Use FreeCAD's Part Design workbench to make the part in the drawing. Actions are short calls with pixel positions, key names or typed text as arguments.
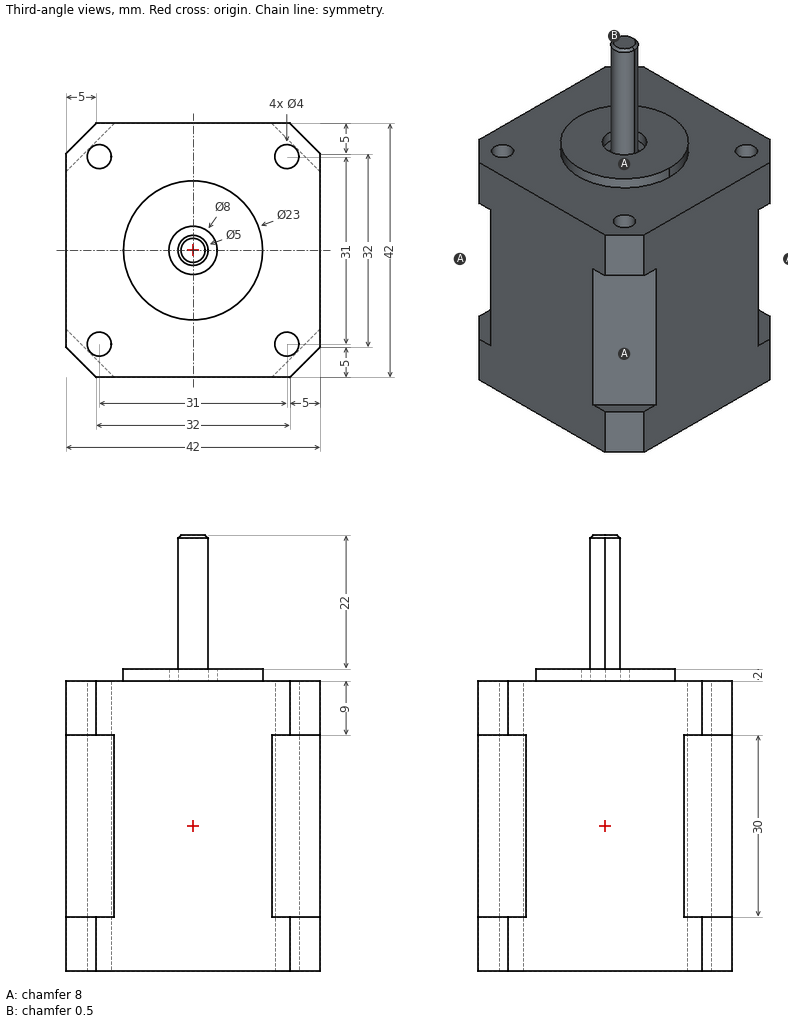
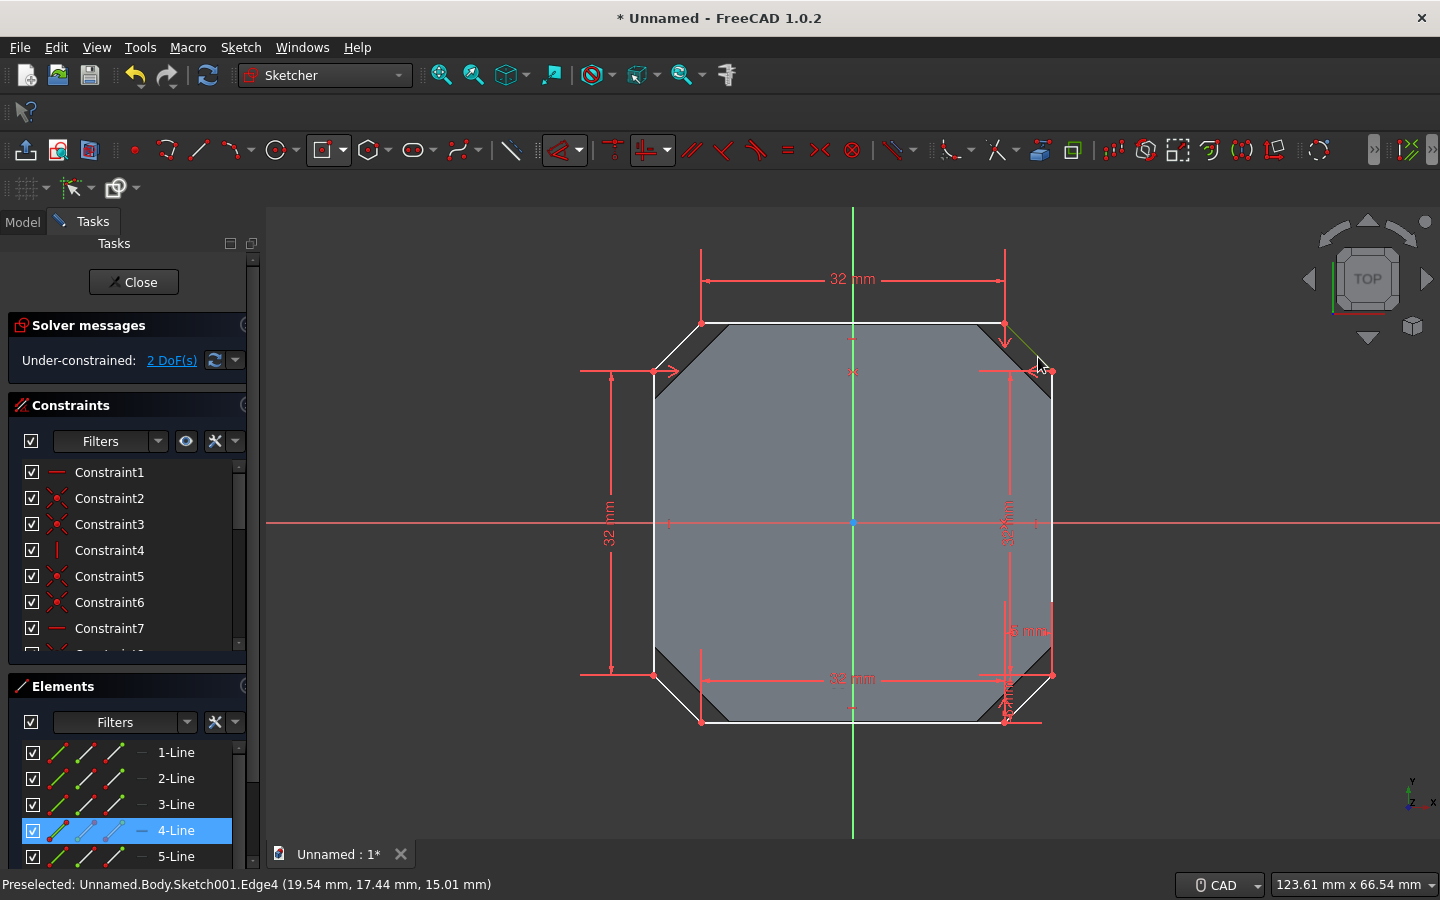
click(582, 150)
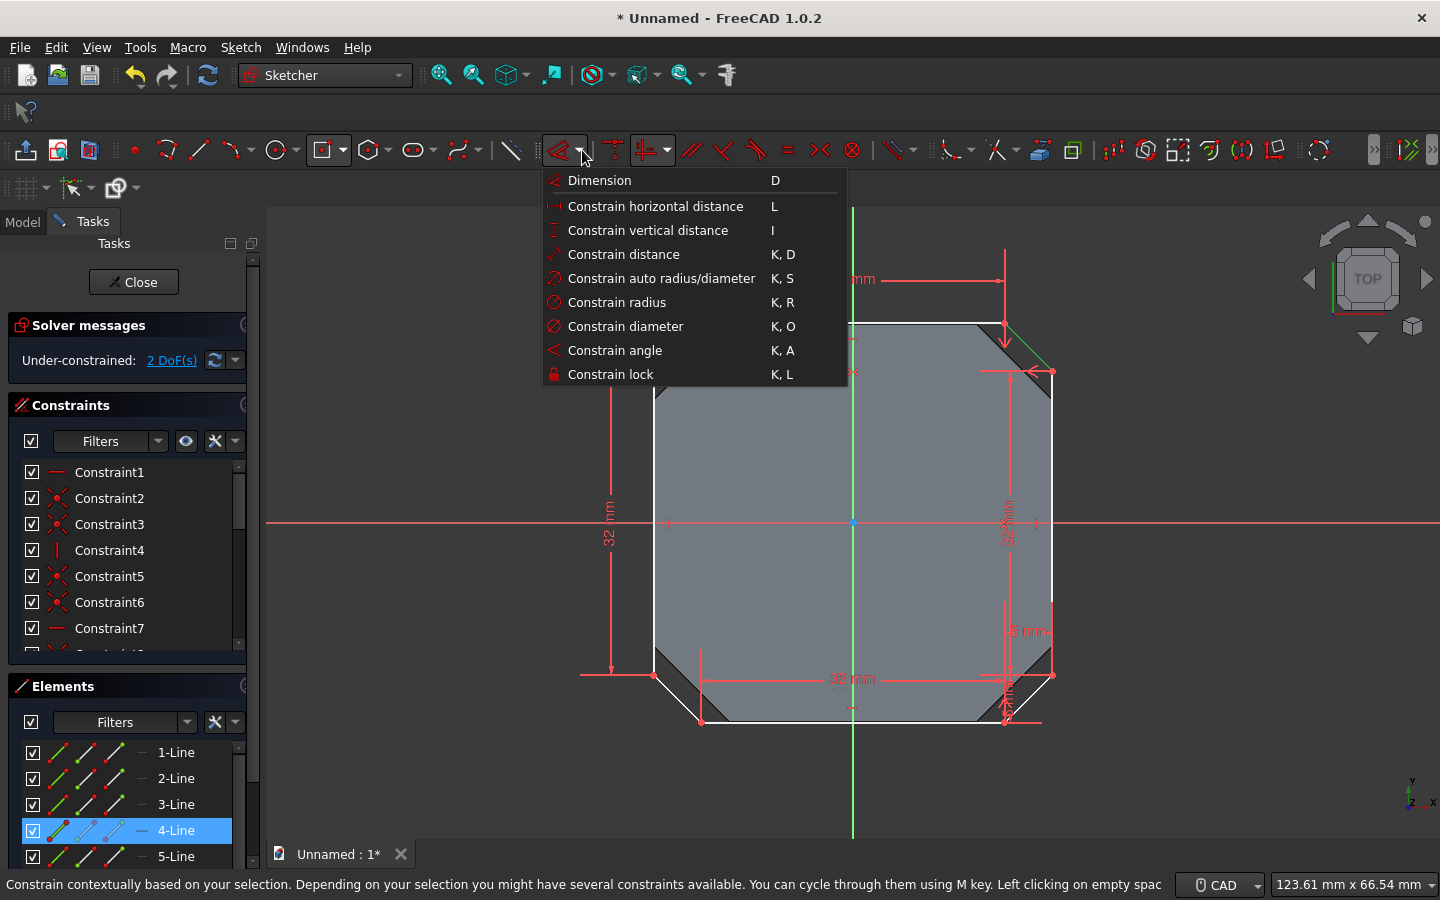
click(695, 230)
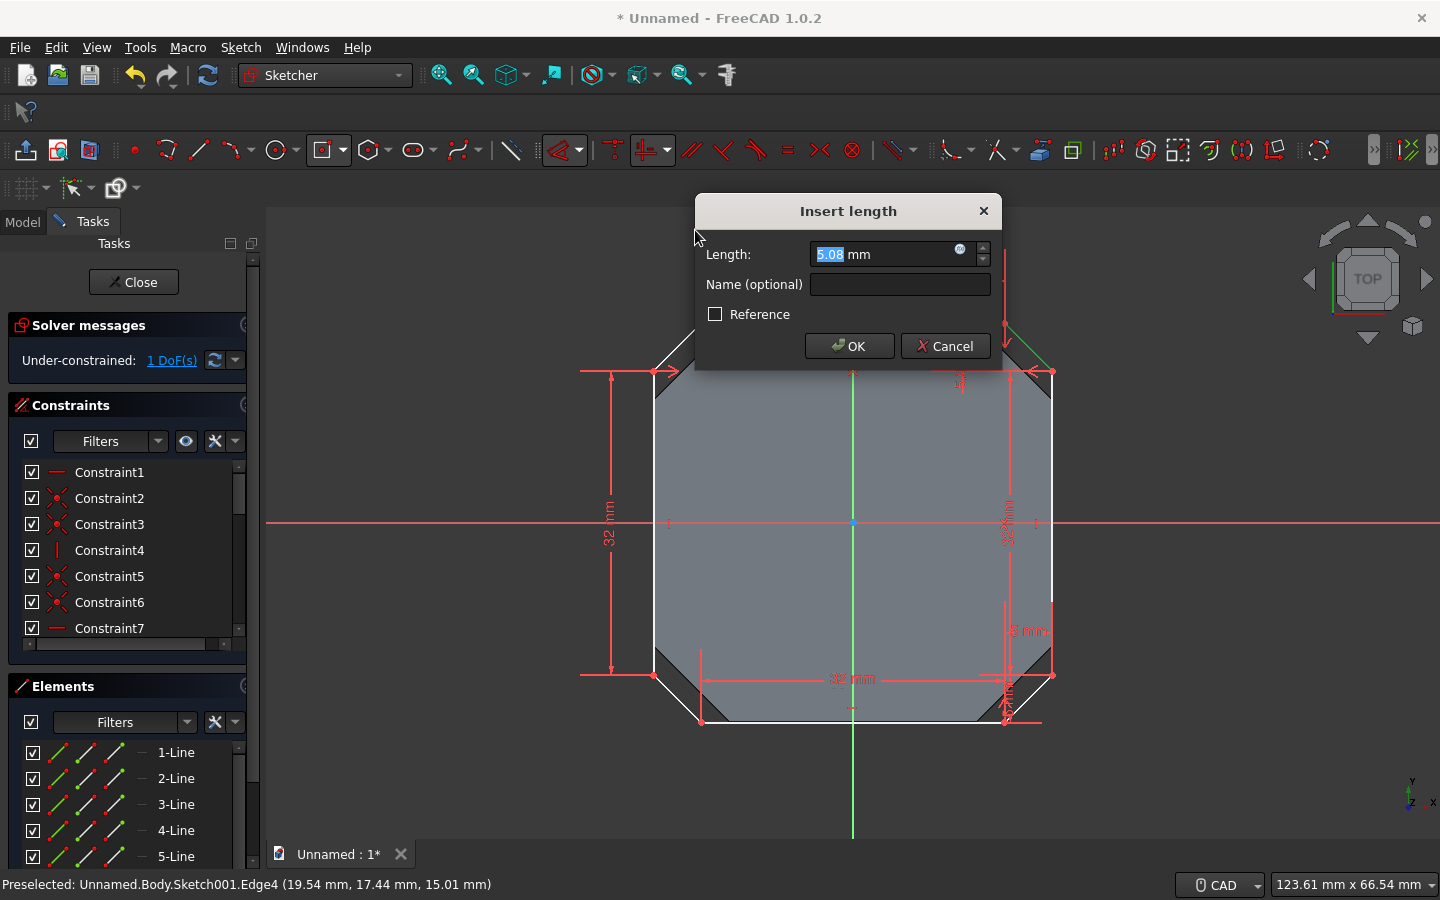
text(5)
key(Return)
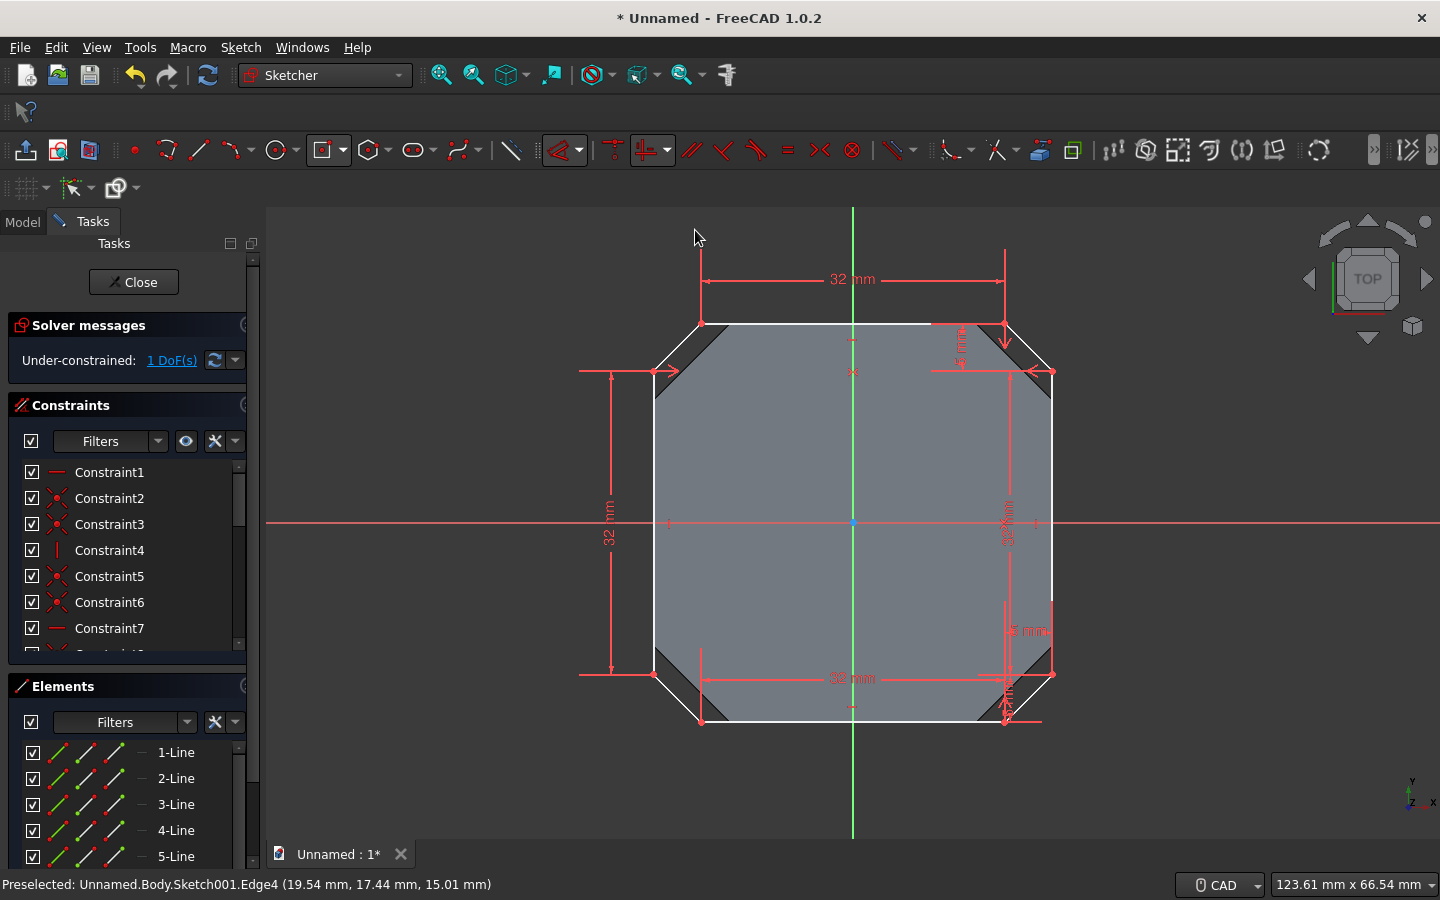
click(687, 338)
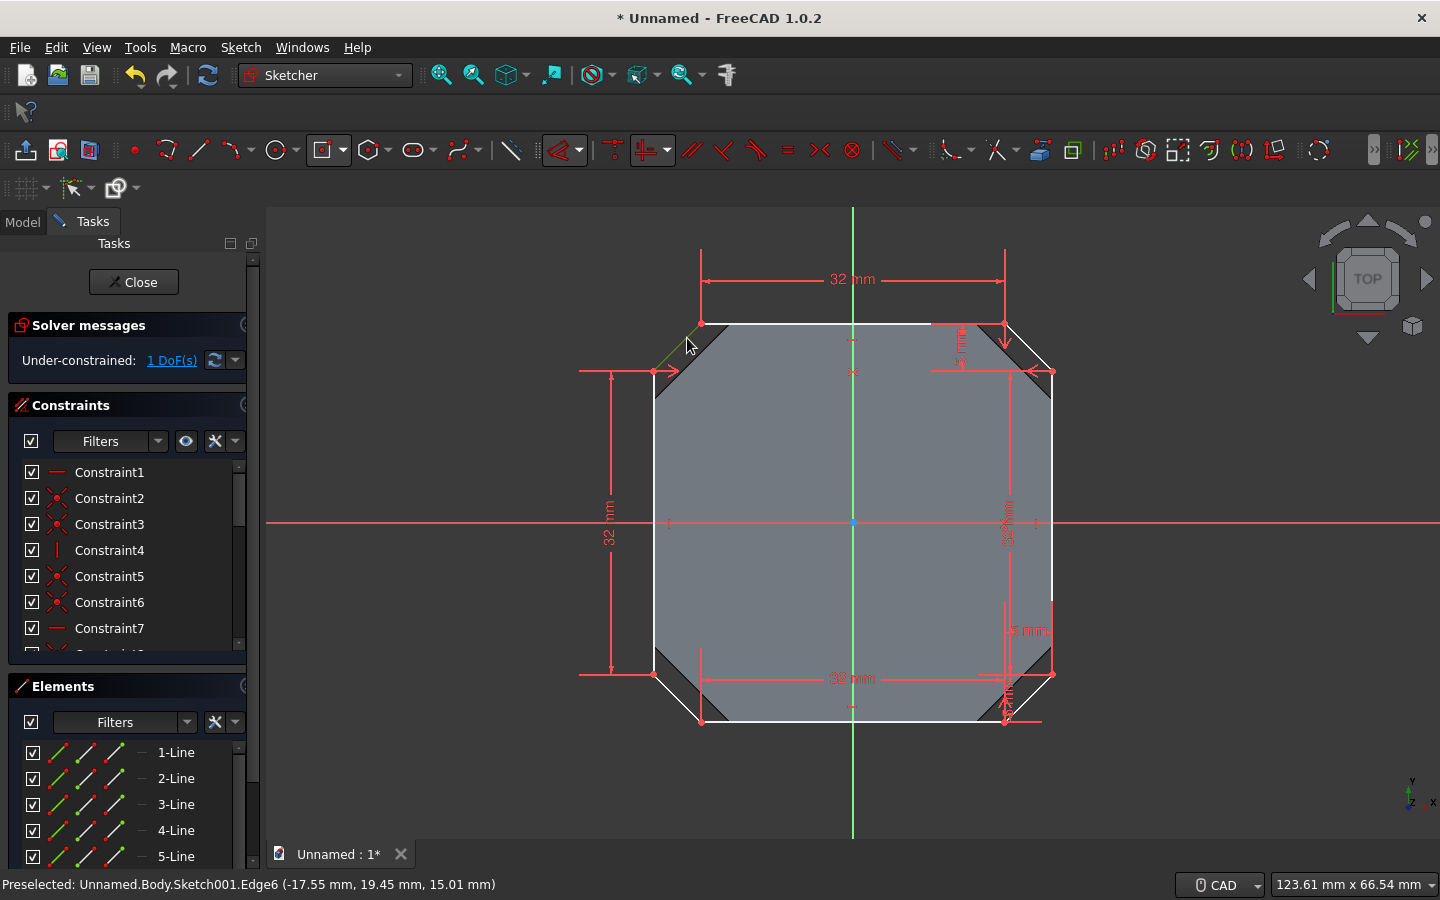
click(582, 150)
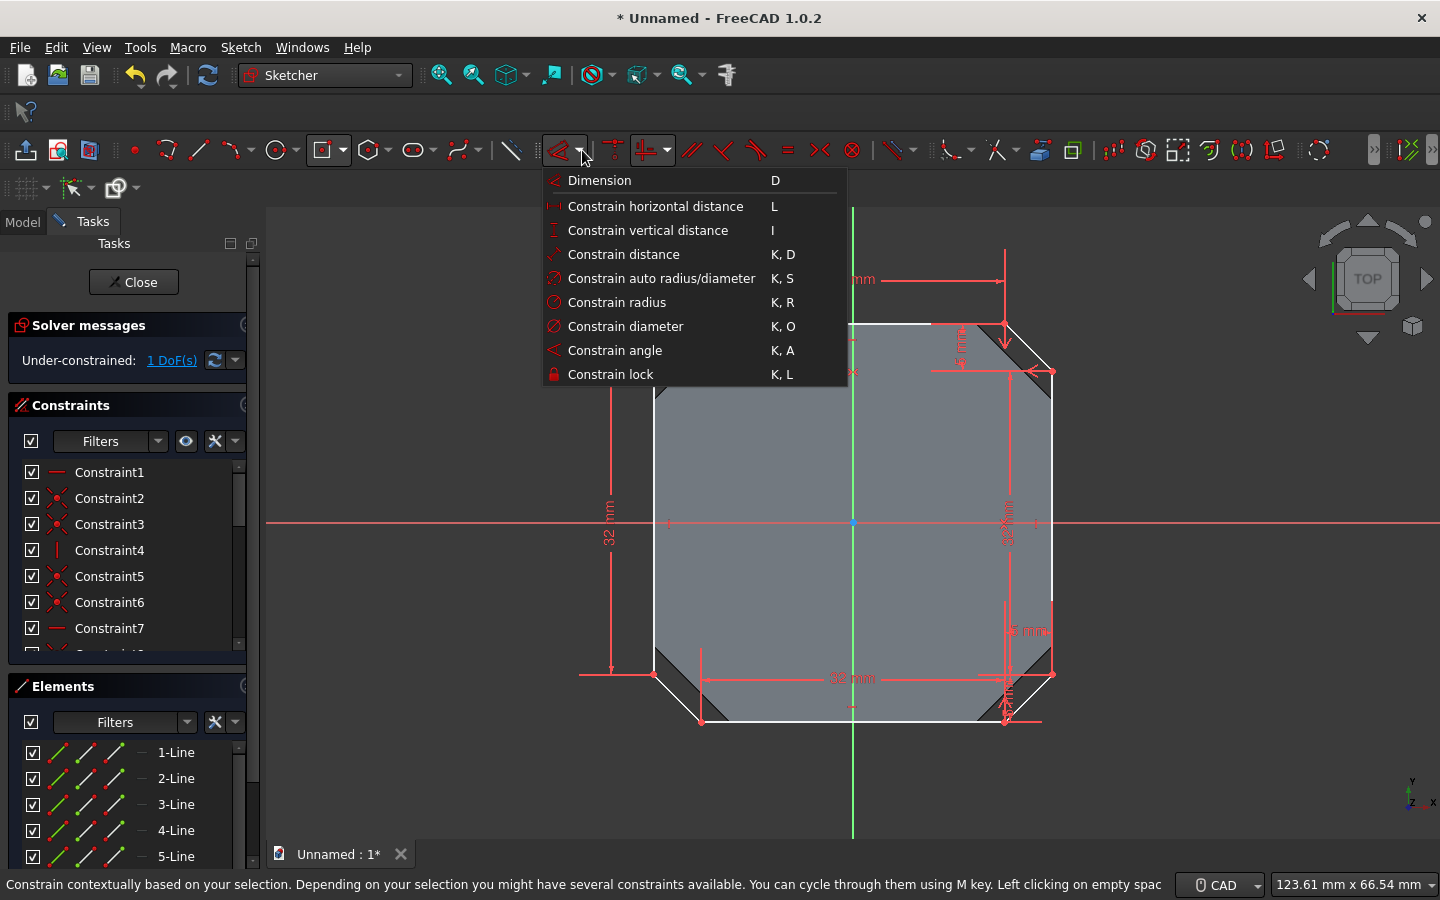
click(695, 206)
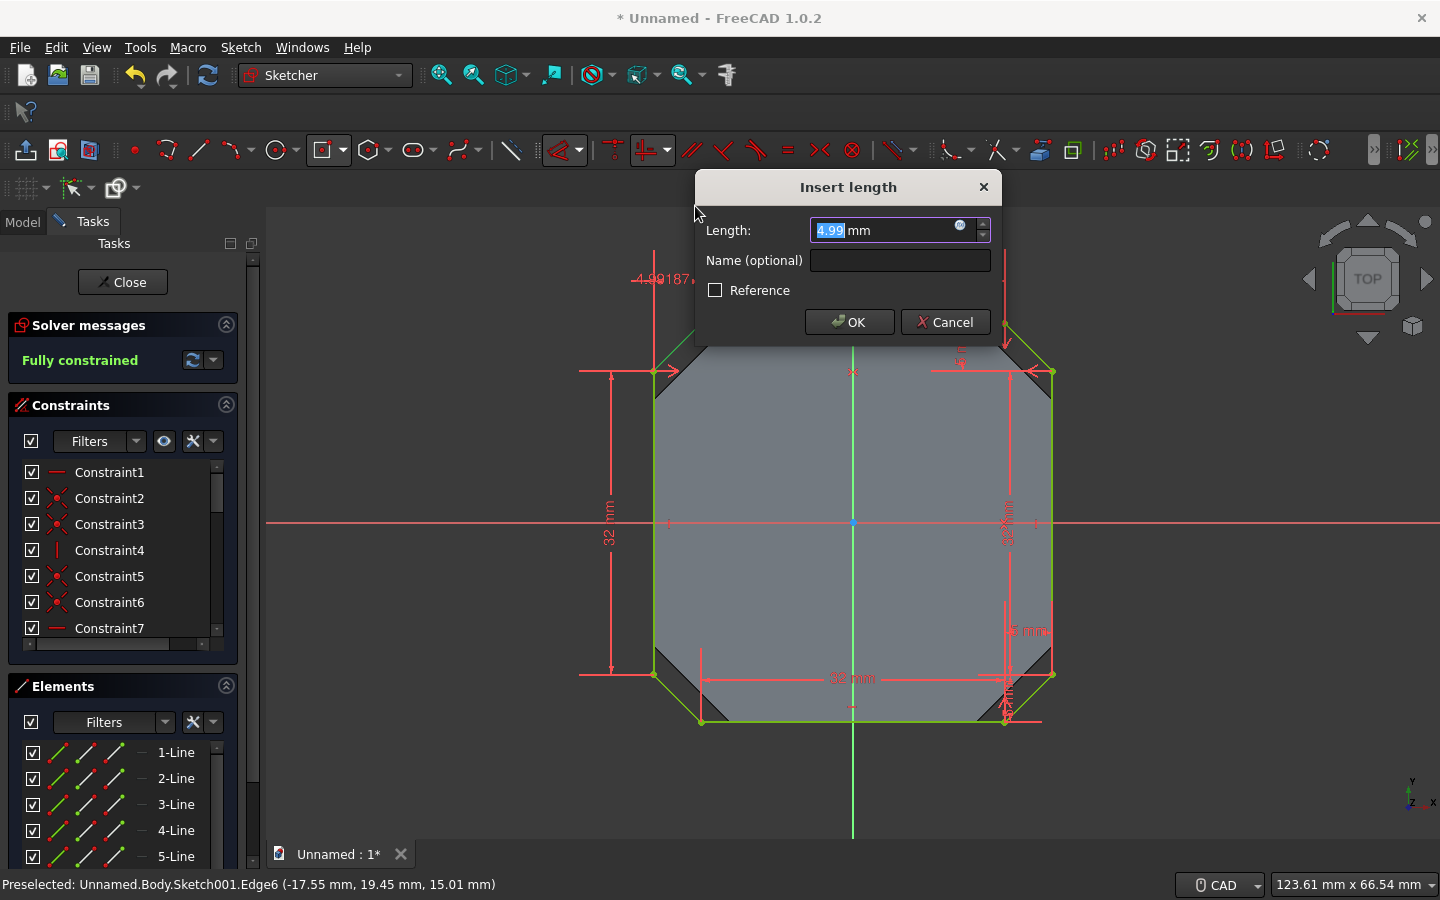
text(5)
key(Return)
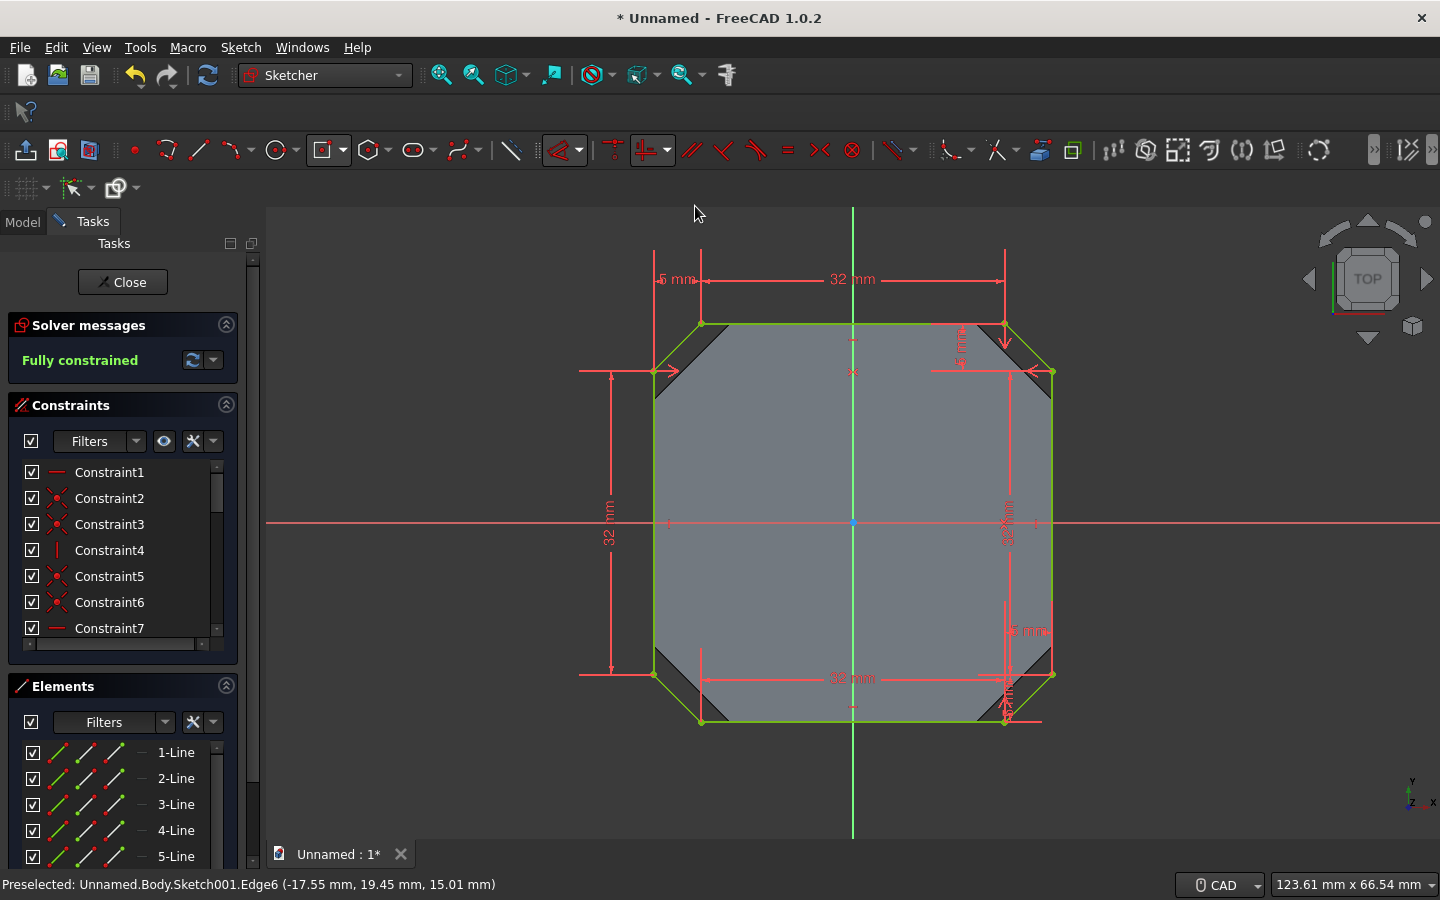
click(123, 282)